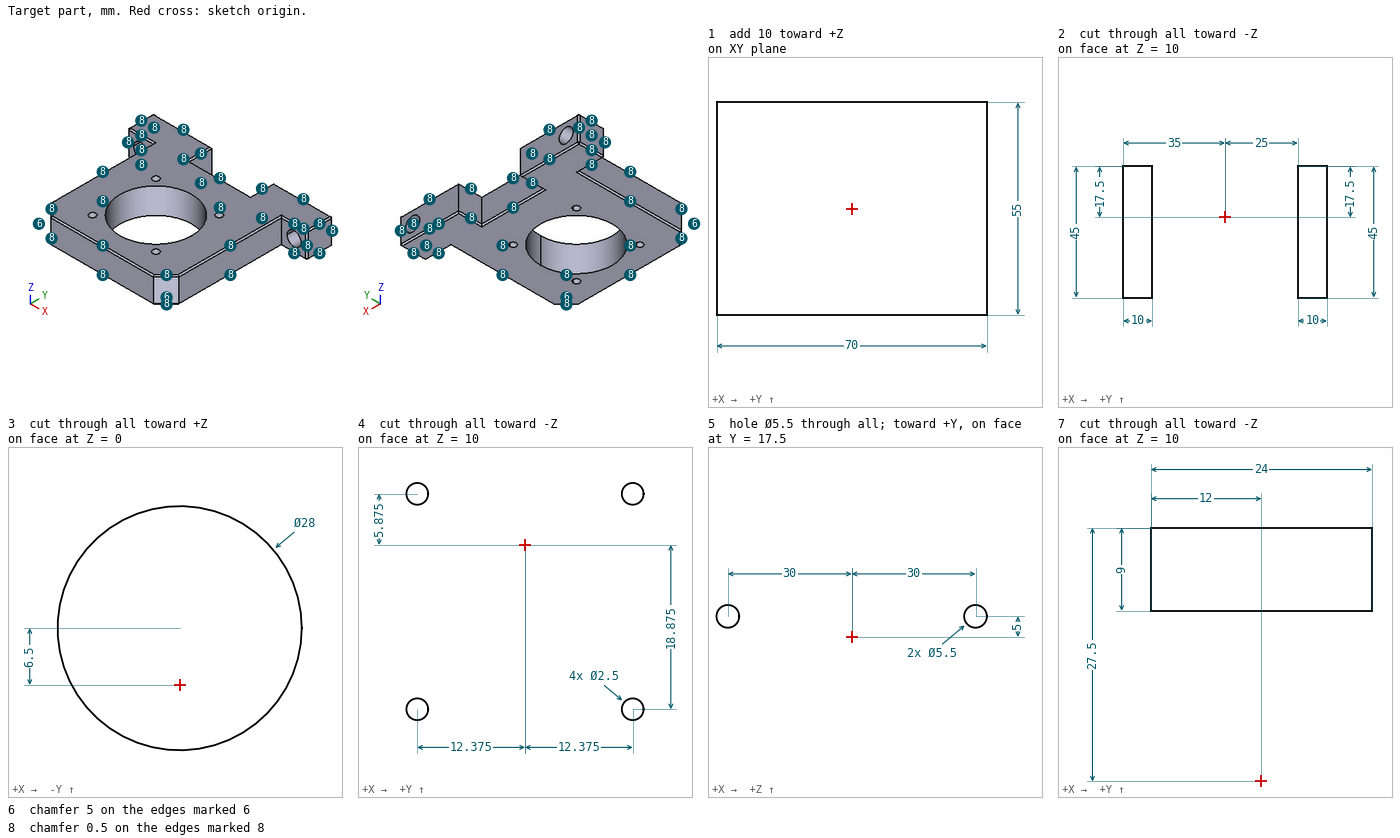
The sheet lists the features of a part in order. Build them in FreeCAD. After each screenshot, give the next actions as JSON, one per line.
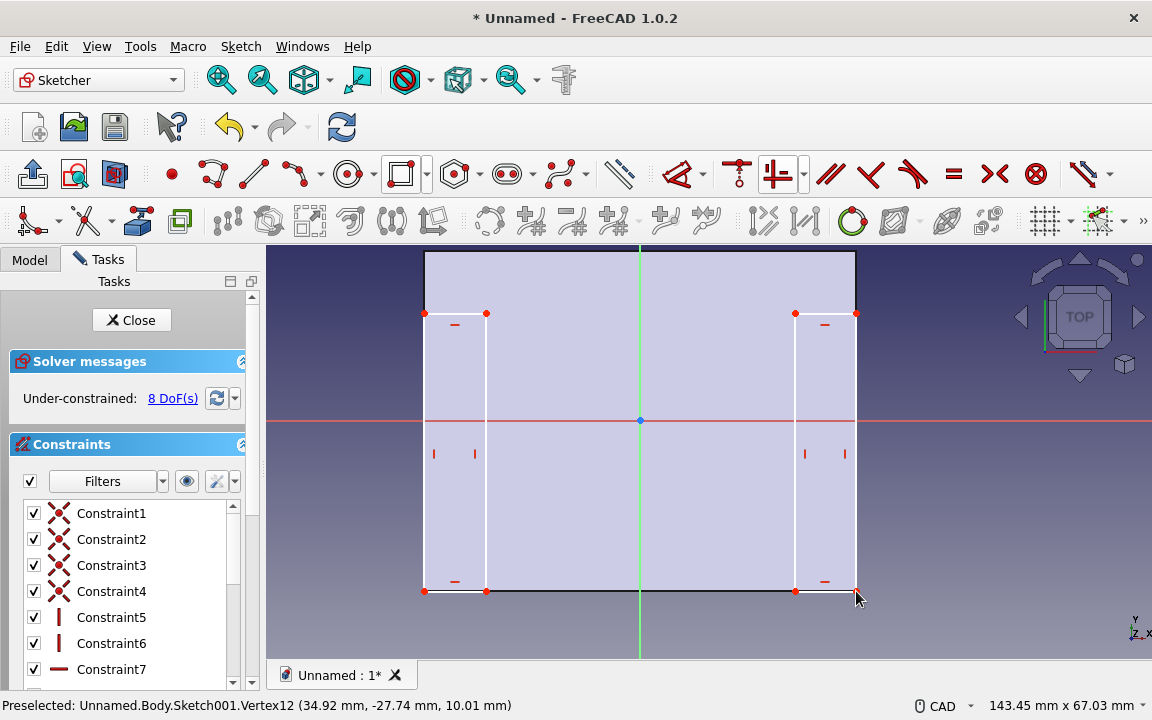
{"action": "left_click", "coordinate": [424, 397]}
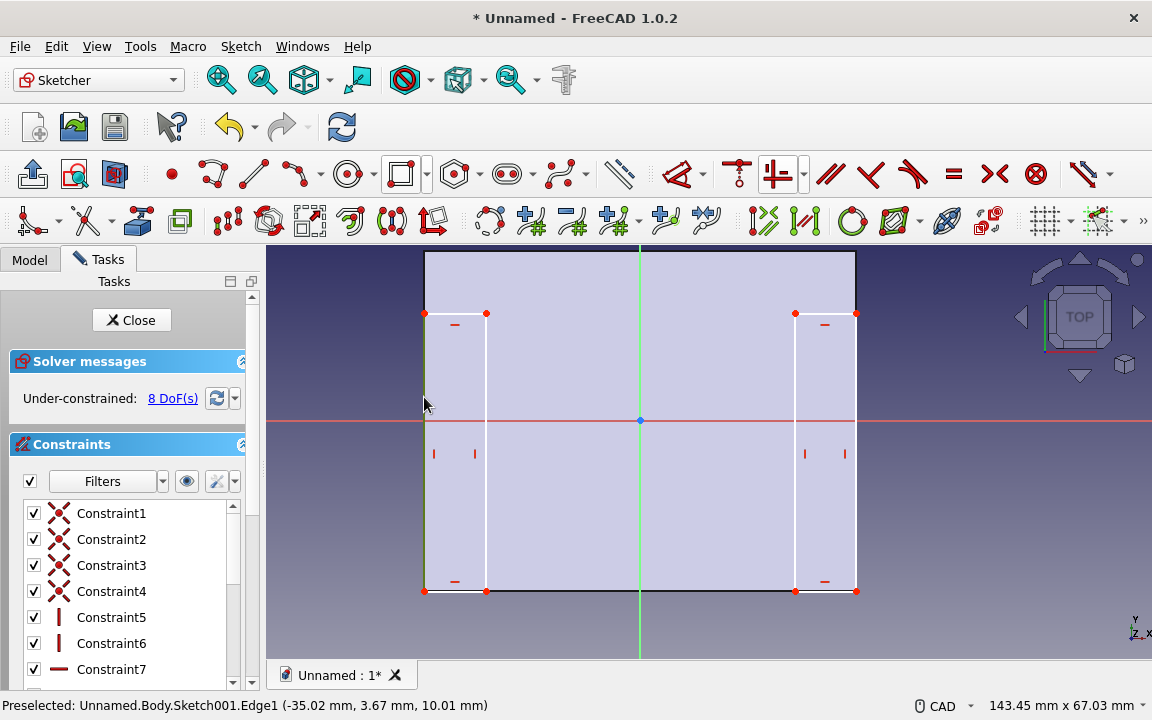
{"action": "left_click", "coordinate": [702, 174]}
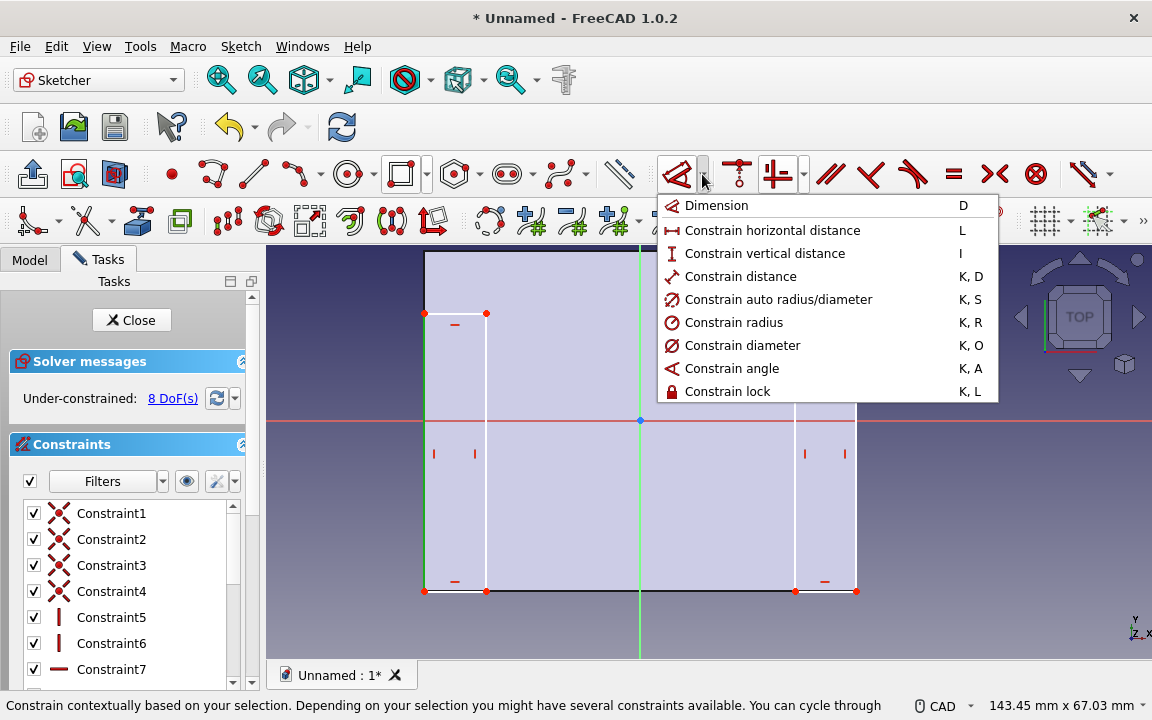
{"action": "left_click", "coordinate": [828, 254]}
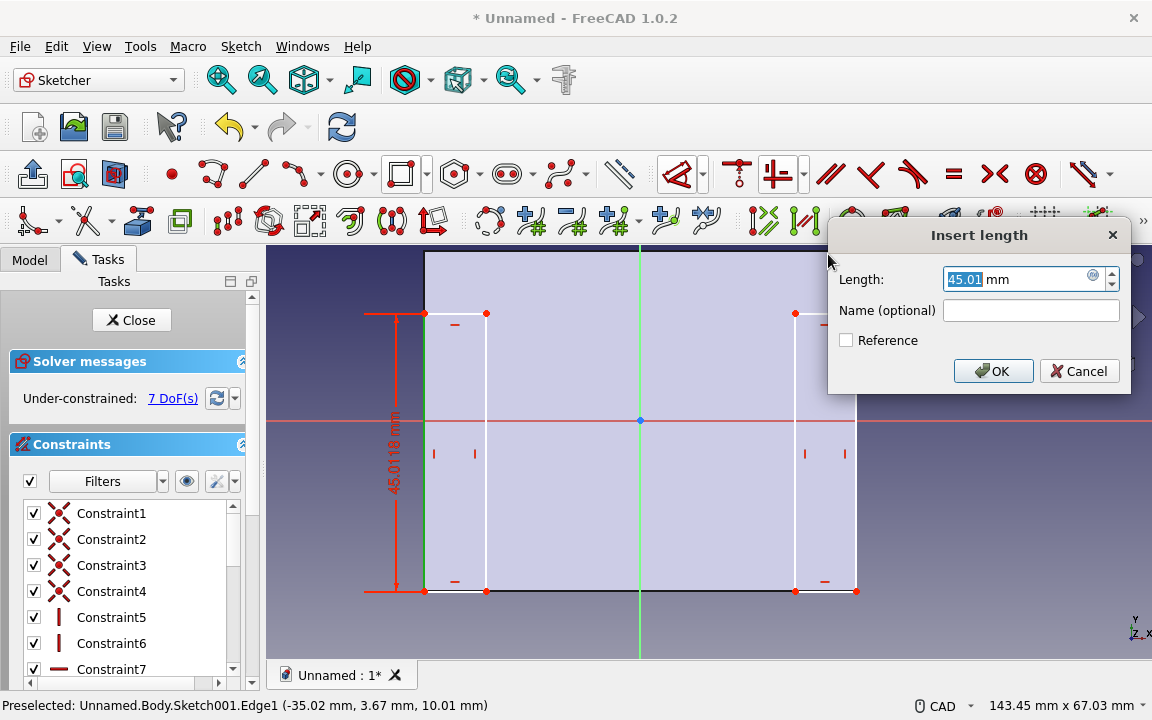
{"action": "type", "text": "45"}
{"action": "key", "text": "Return"}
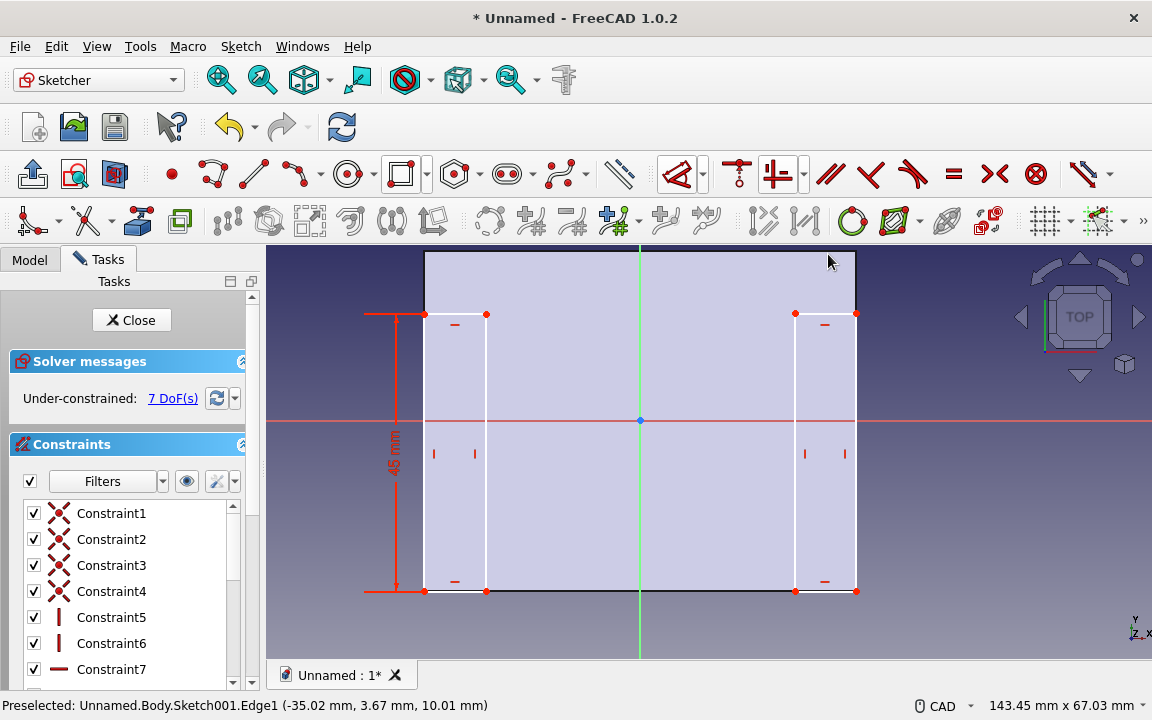
{"action": "left_click", "coordinate": [443, 592]}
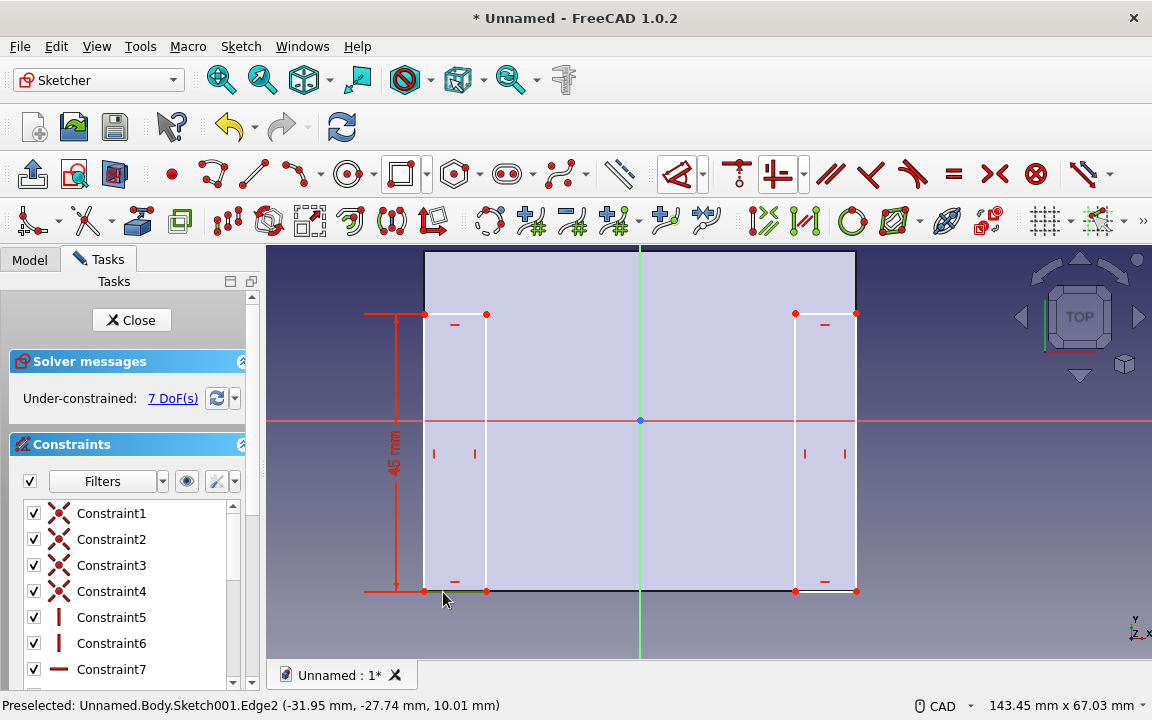
{"action": "key", "text": "l"}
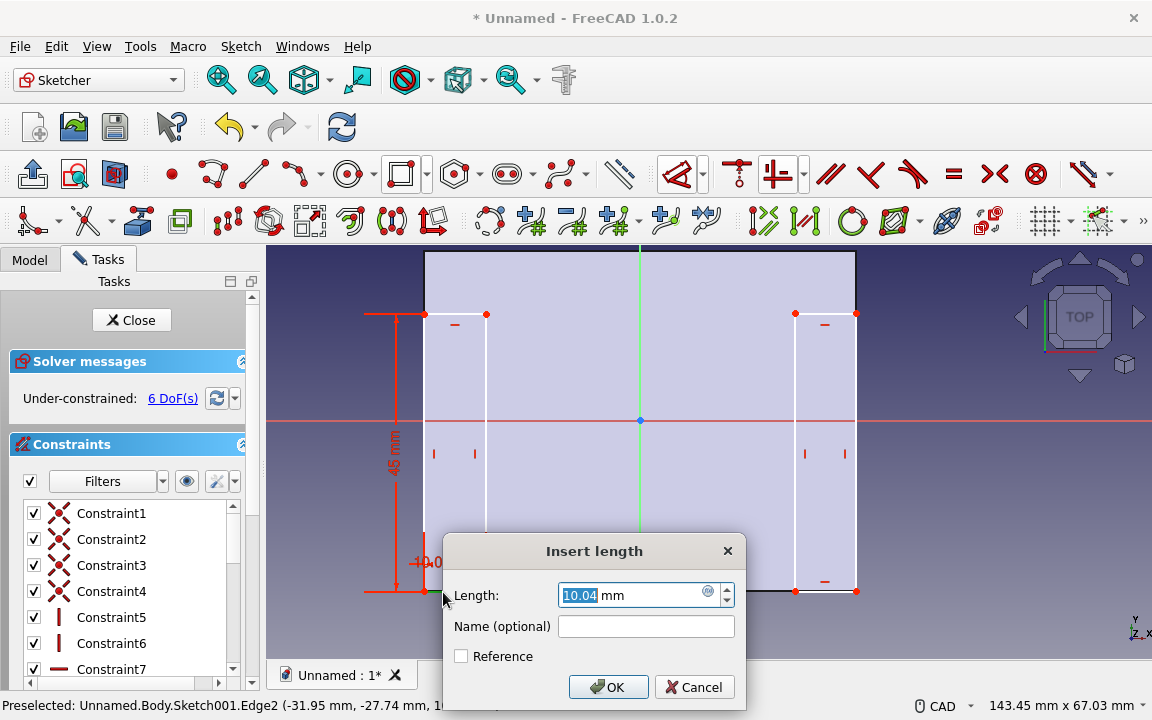
{"action": "type", "text": "10"}
{"action": "key", "text": "Return"}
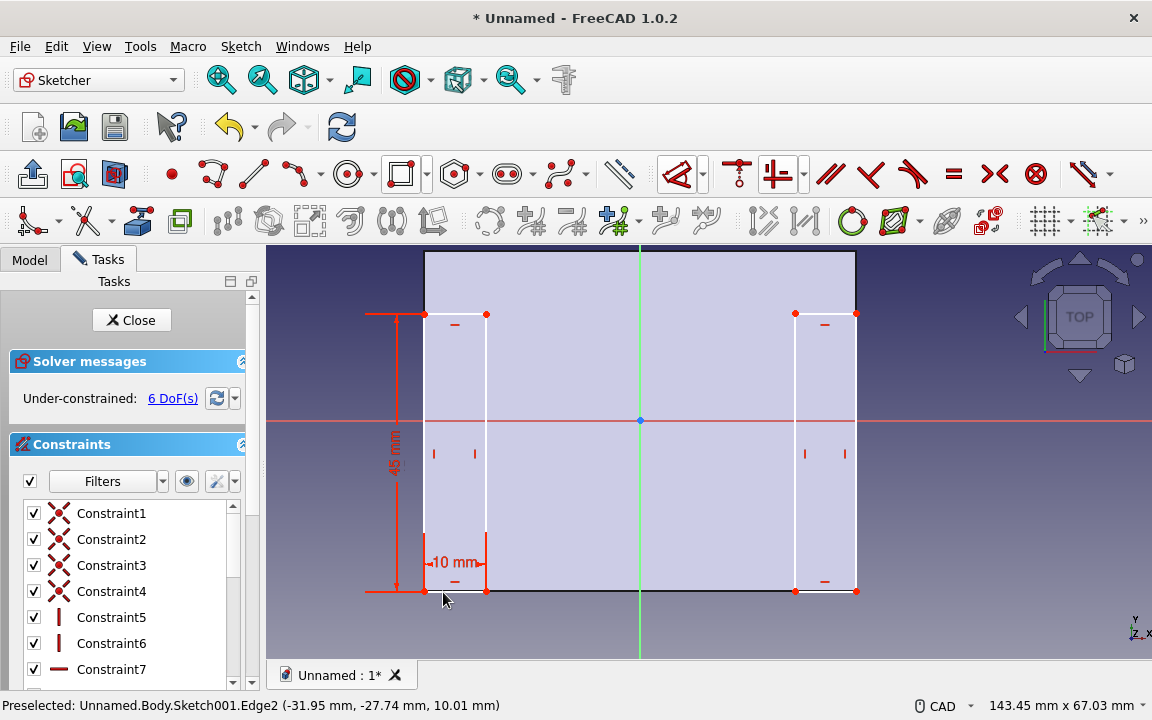
{"action": "left_click", "coordinate": [795, 397]}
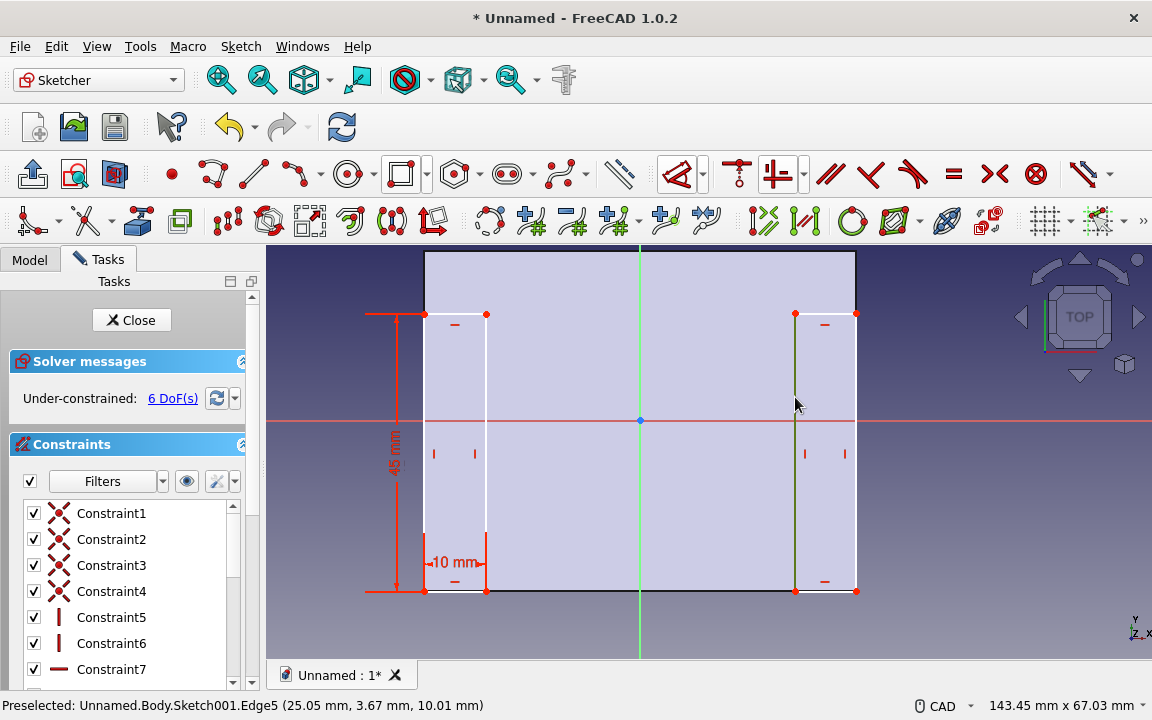
{"action": "left_click", "coordinate": [702, 174]}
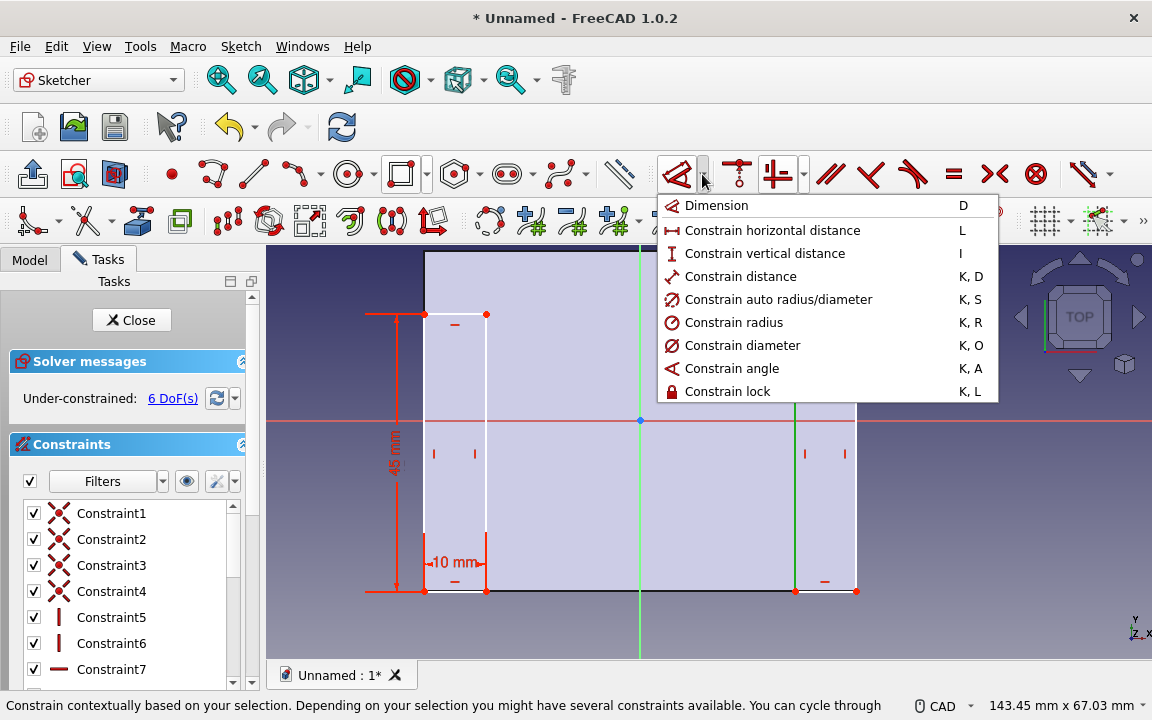
{"action": "left_click", "coordinate": [828, 254]}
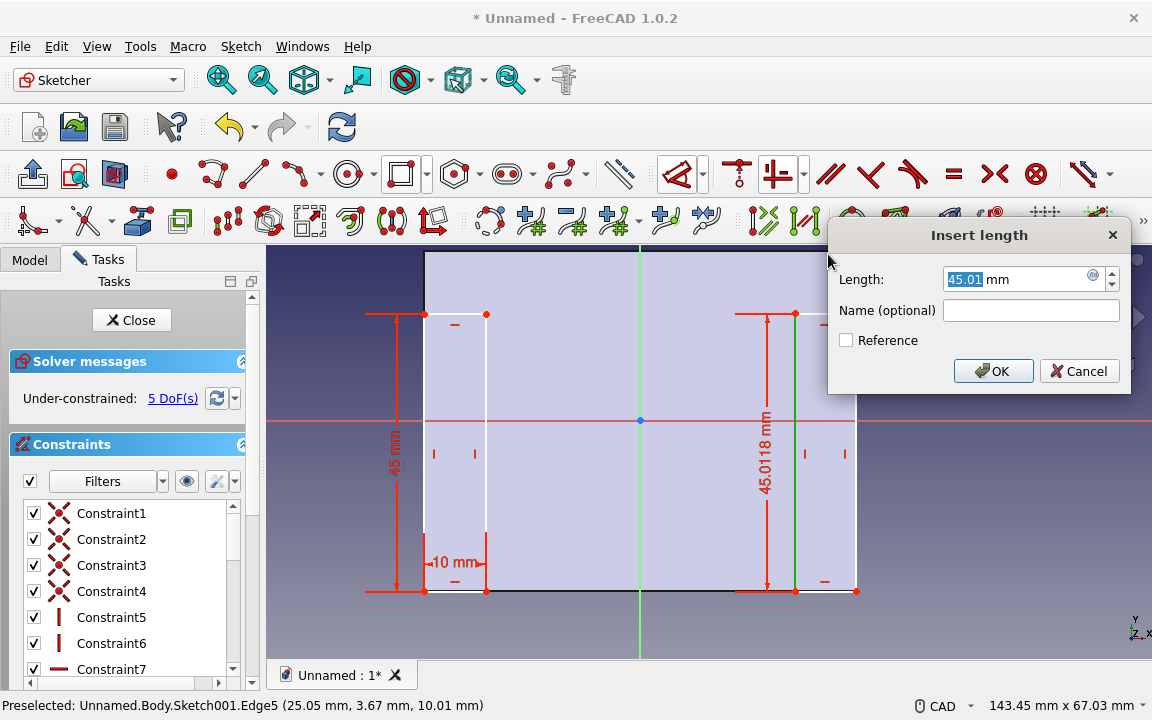
{"action": "type", "text": "45"}
{"action": "key", "text": "Return"}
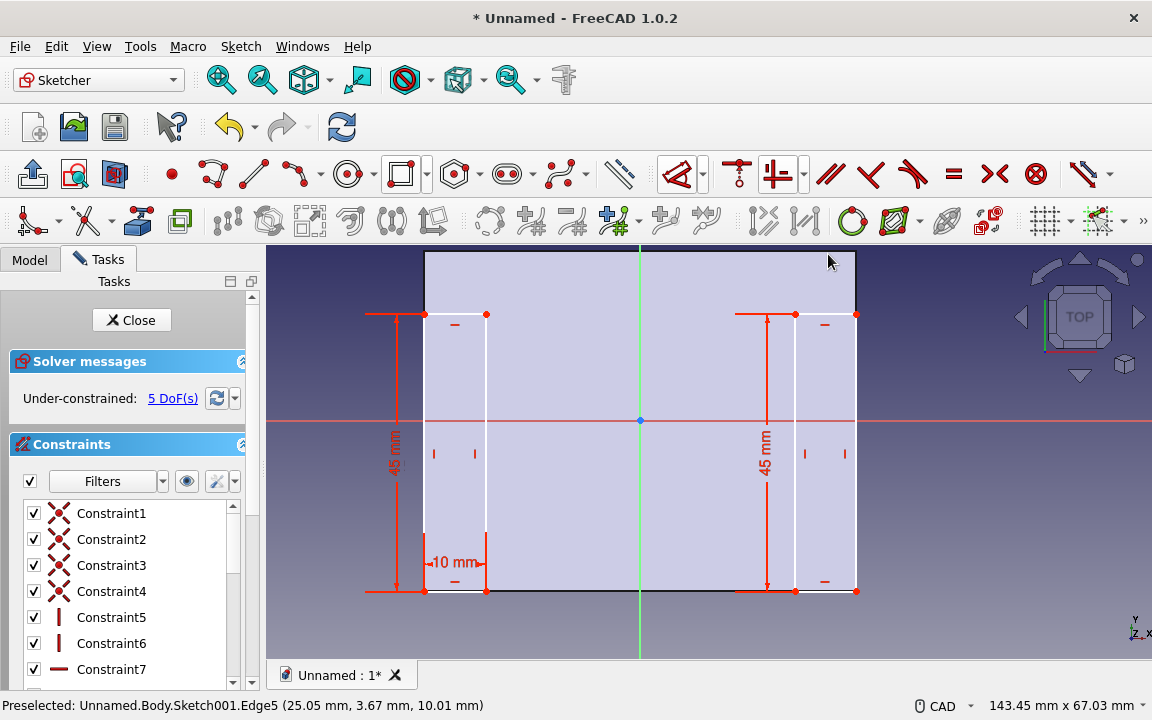
{"action": "left_click", "coordinate": [813, 592]}